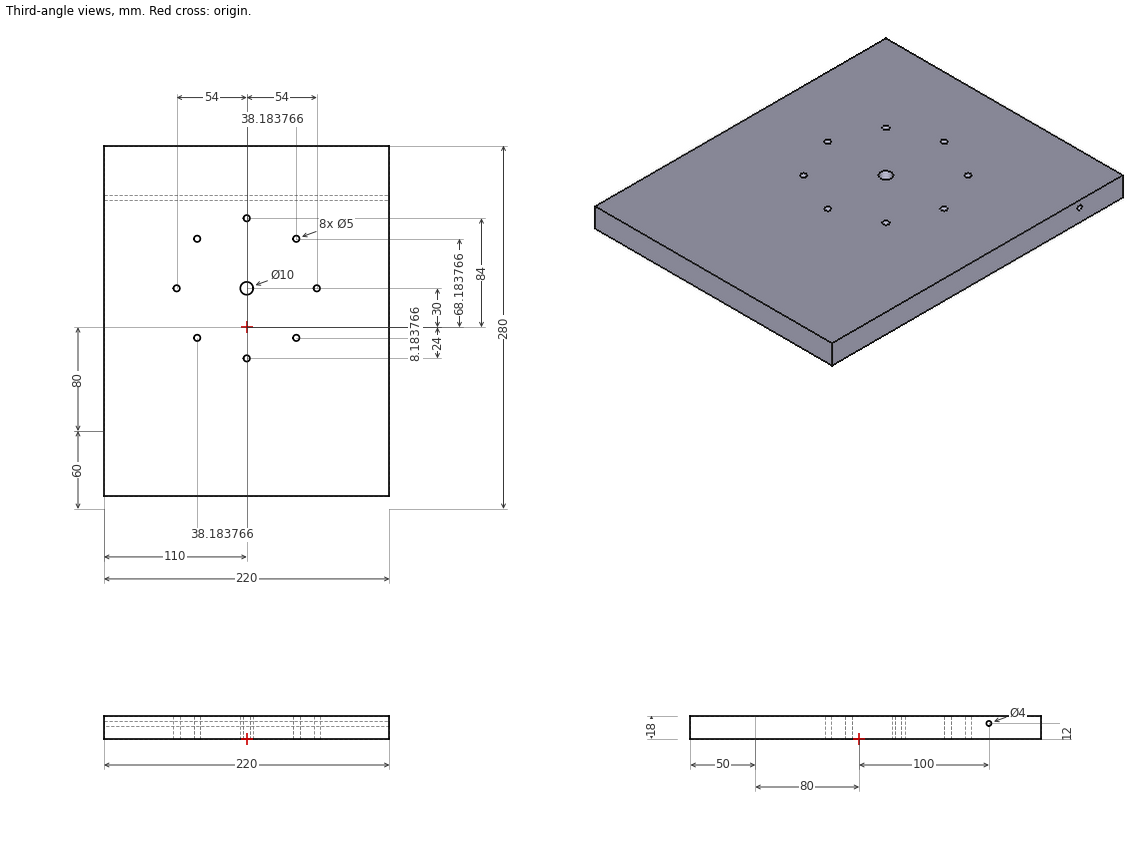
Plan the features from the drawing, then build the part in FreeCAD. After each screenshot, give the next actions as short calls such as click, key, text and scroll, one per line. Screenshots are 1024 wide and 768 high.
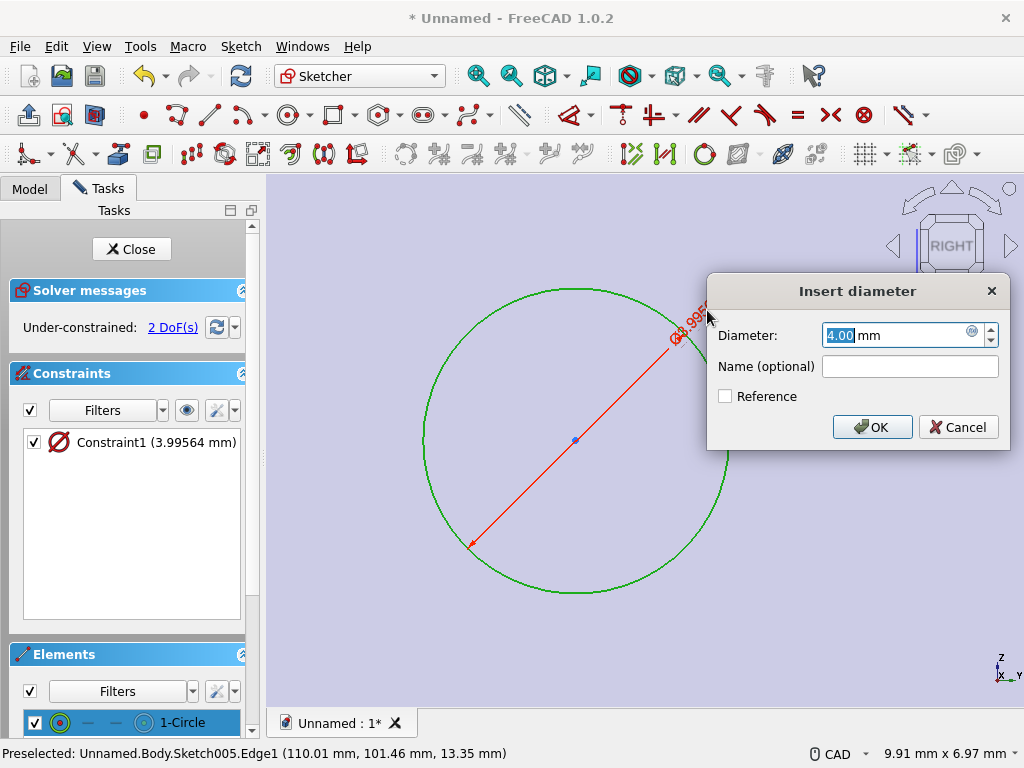
text(4)
key(Return)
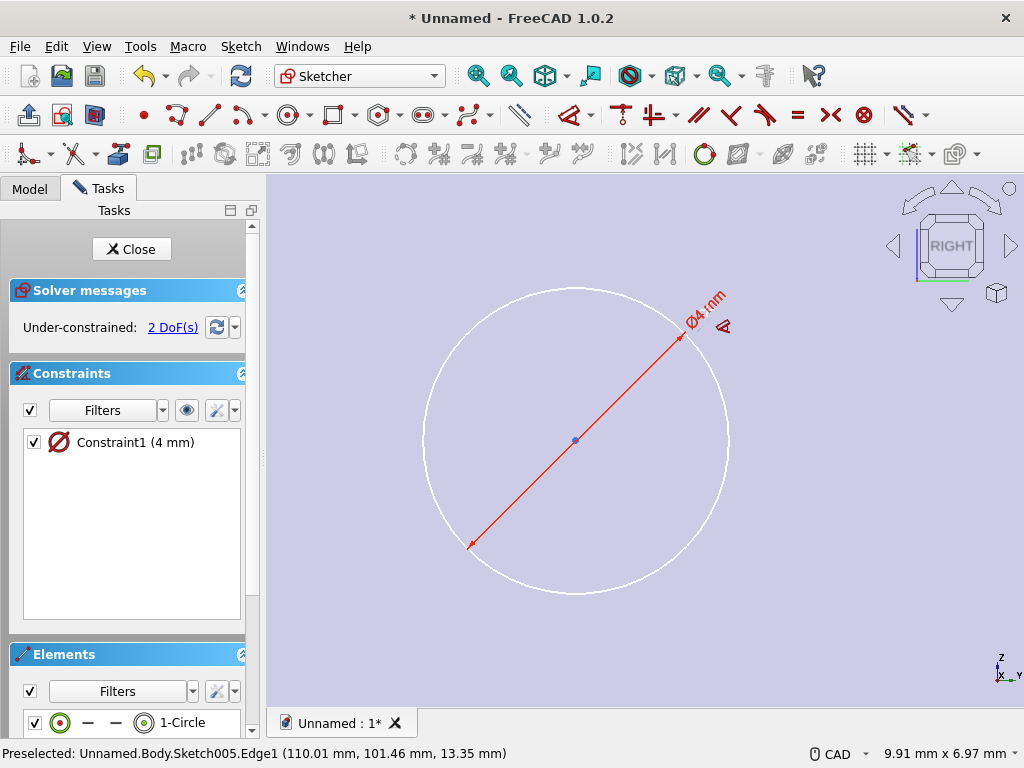
click(576, 441)
click(610, 560)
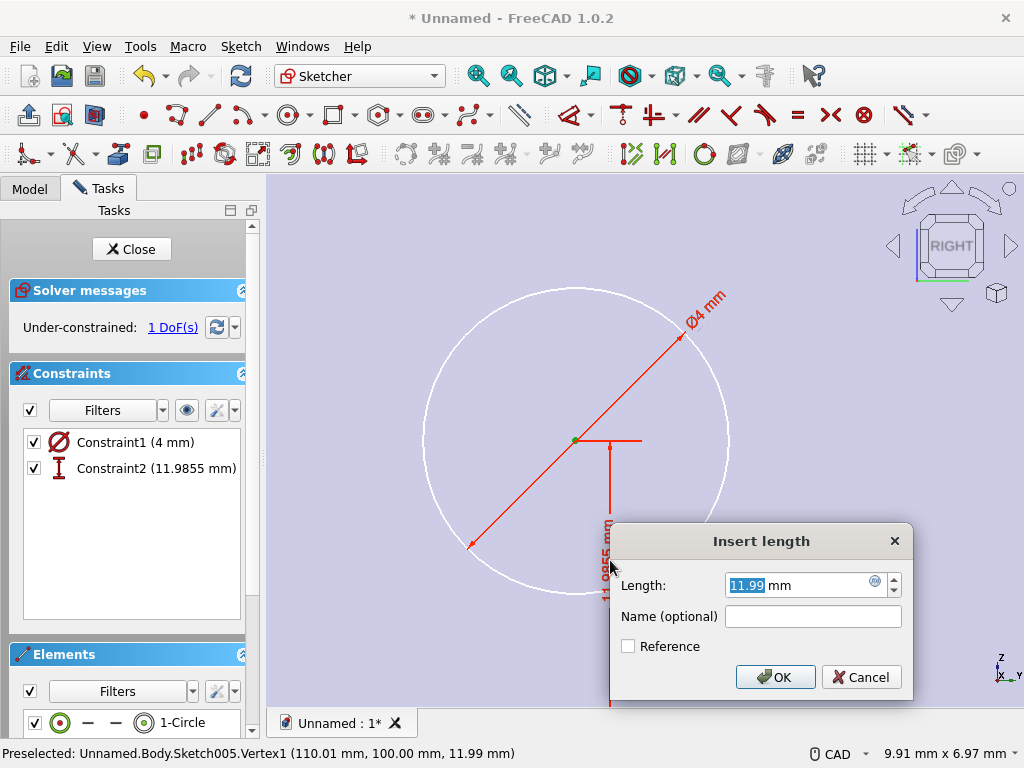
text(12)
key(Return)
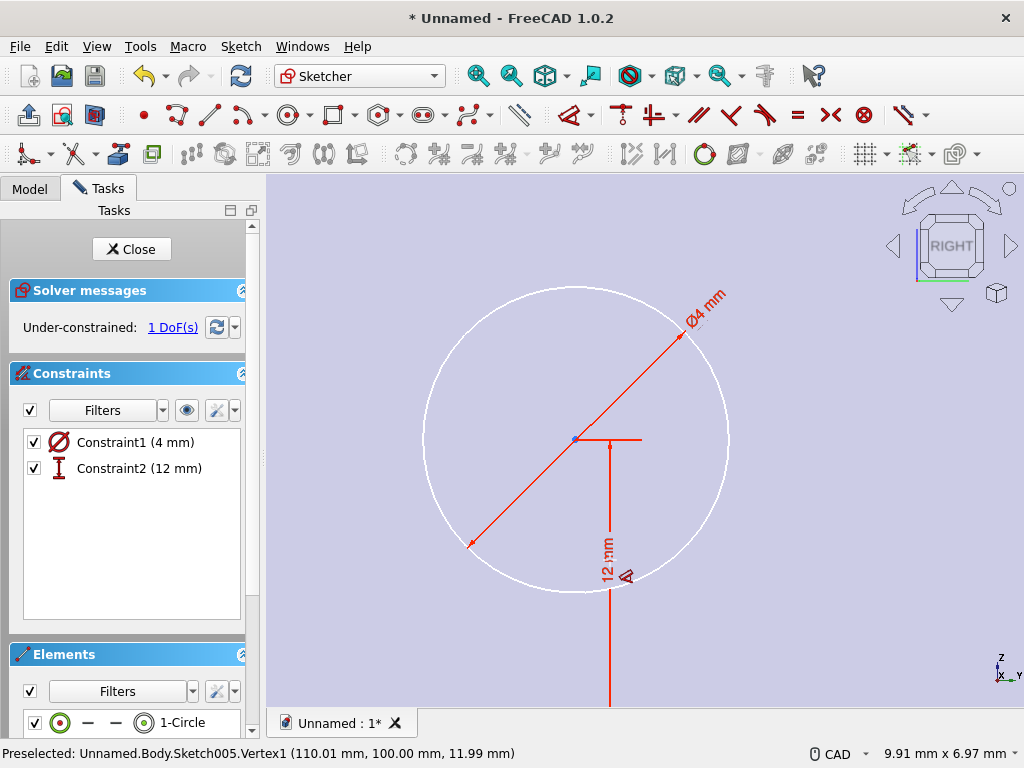
click(576, 440)
click(370, 406)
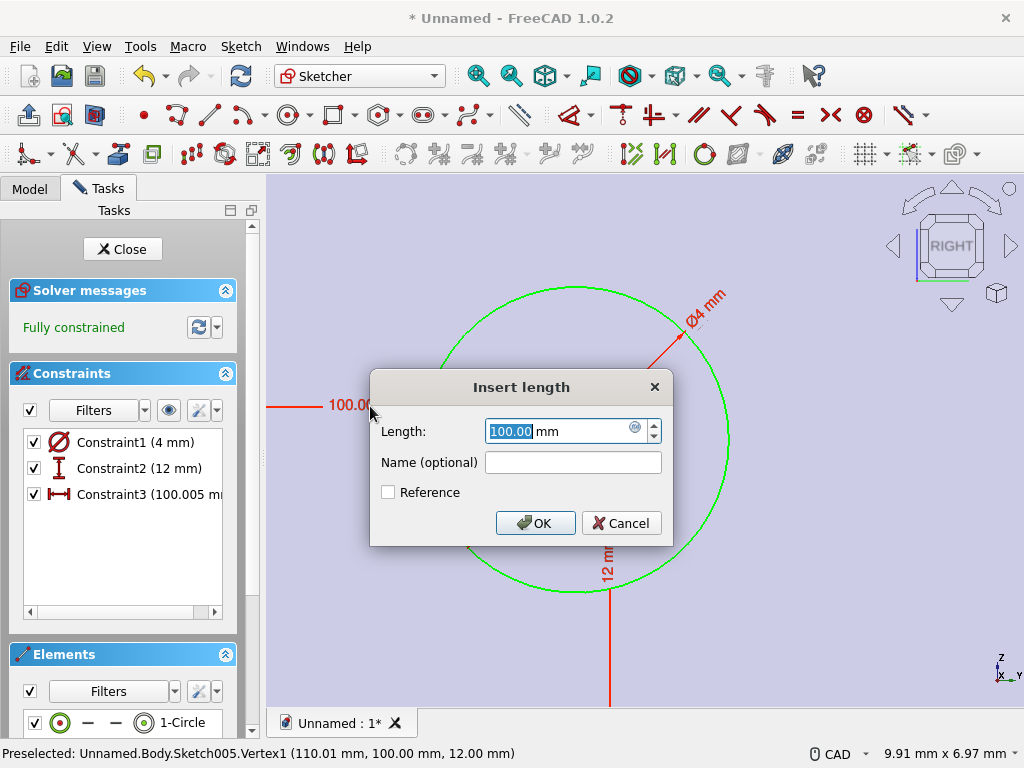
text(100)
key(Return)
key(Escape)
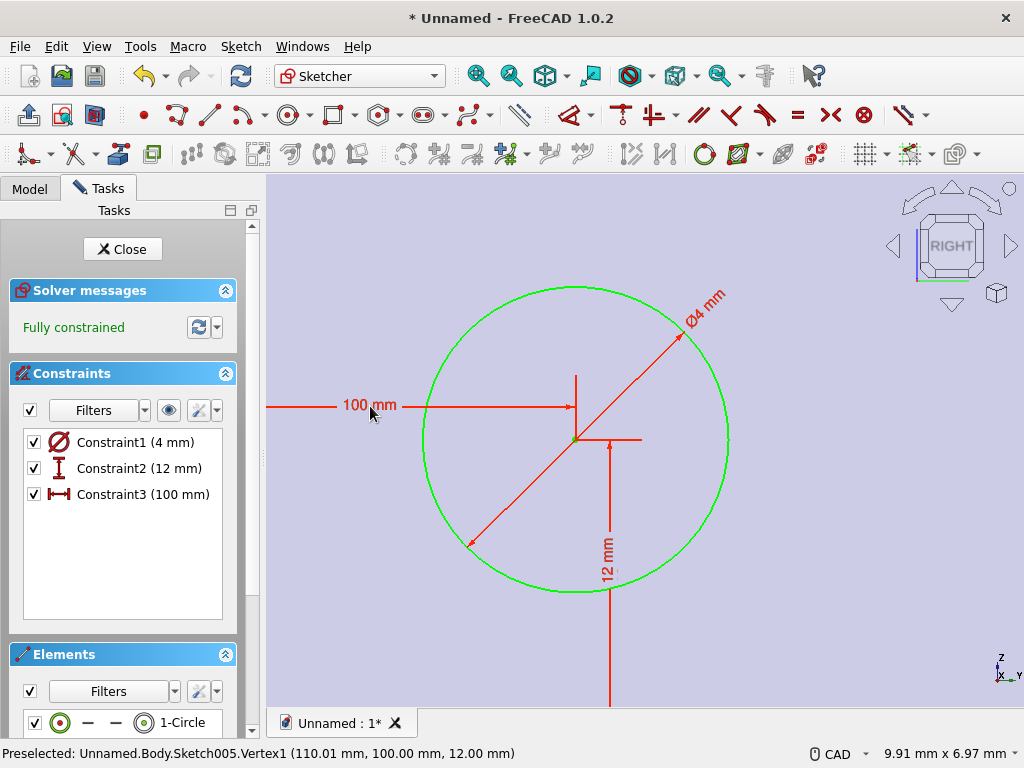
click(123, 249)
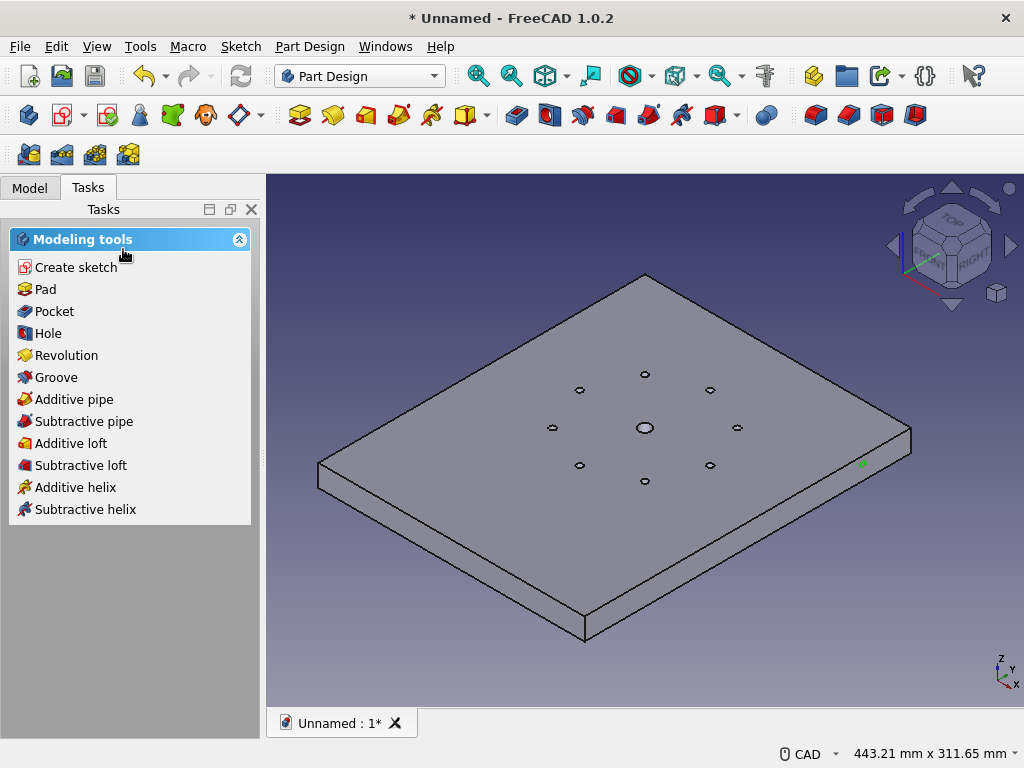
click(517, 116)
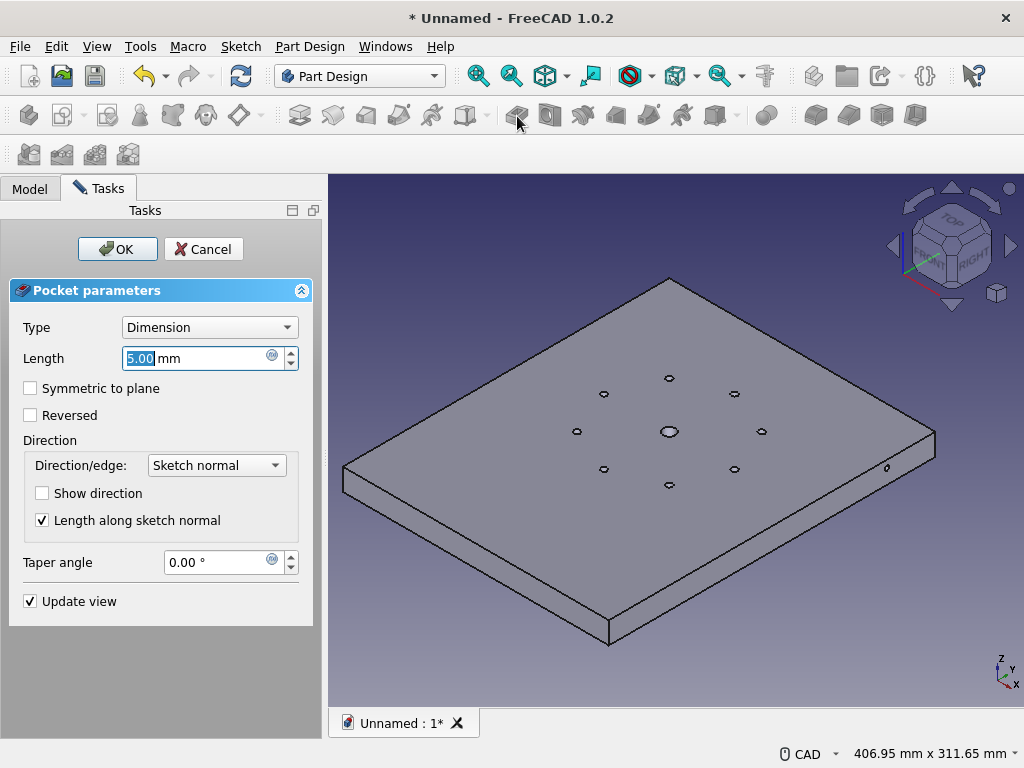
click(210, 328)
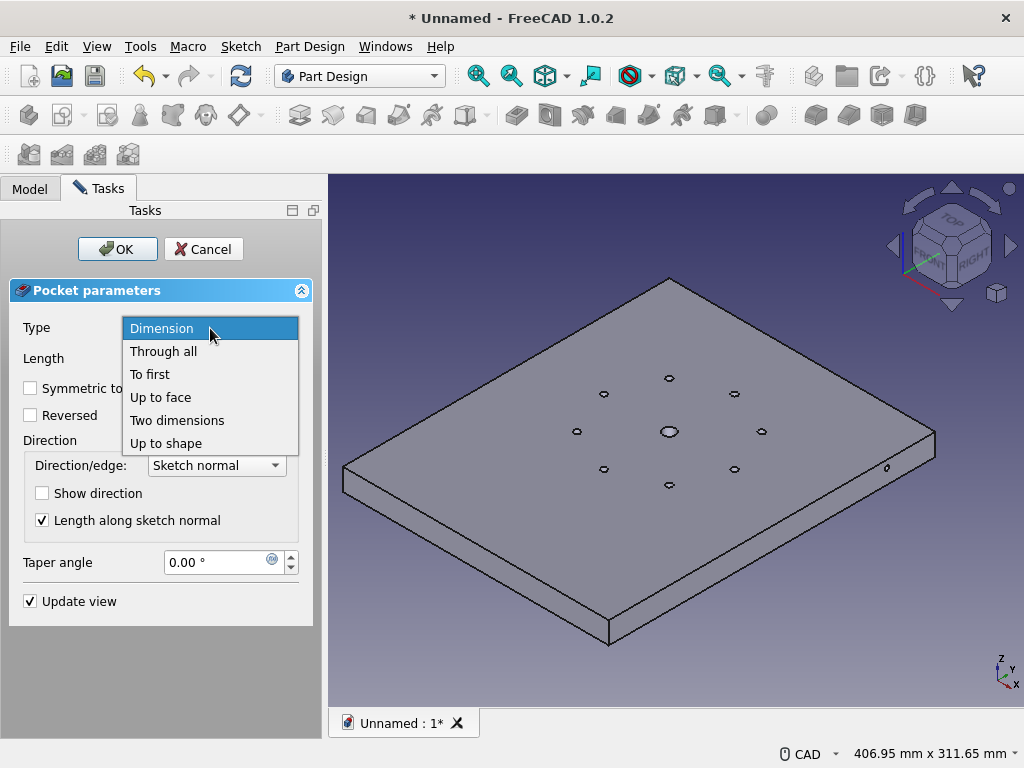
click(208, 352)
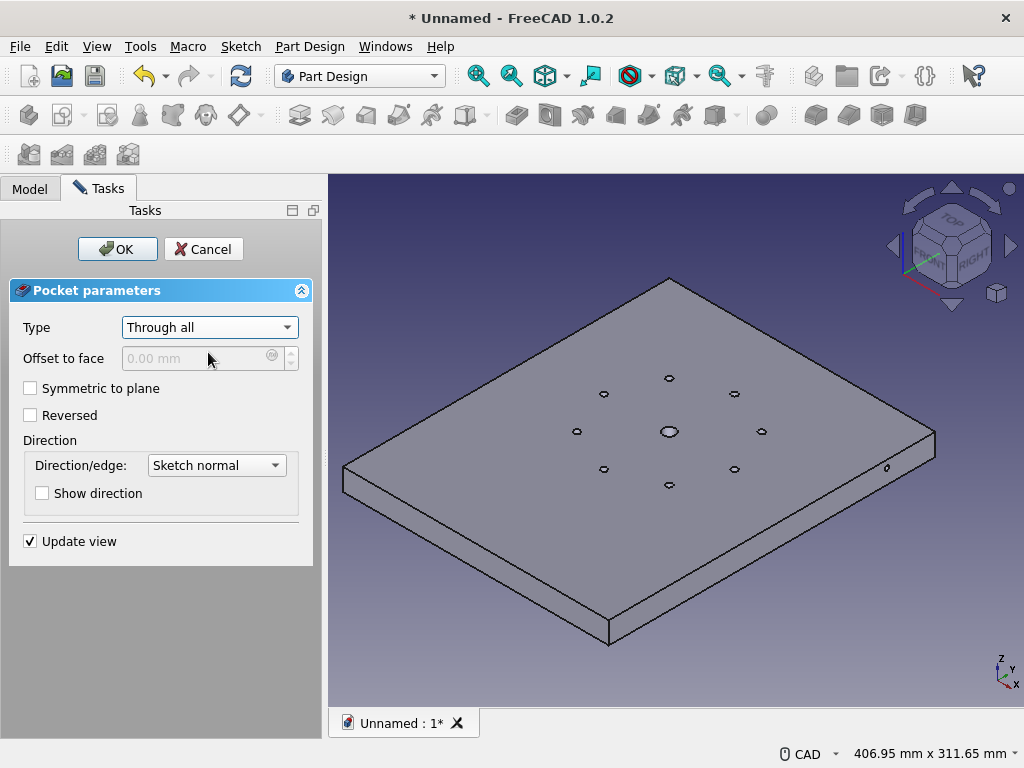
click(118, 249)